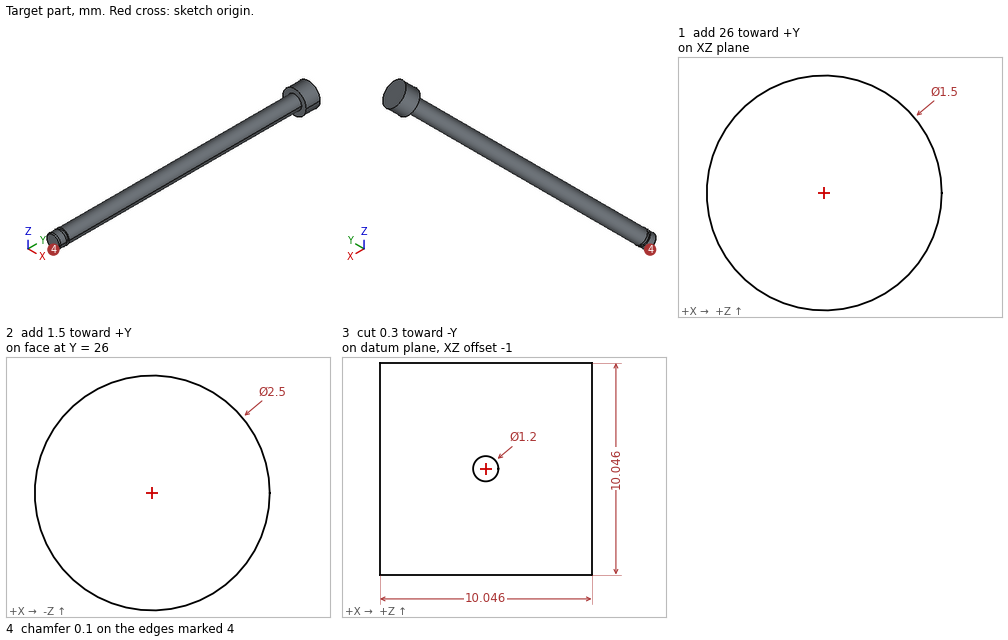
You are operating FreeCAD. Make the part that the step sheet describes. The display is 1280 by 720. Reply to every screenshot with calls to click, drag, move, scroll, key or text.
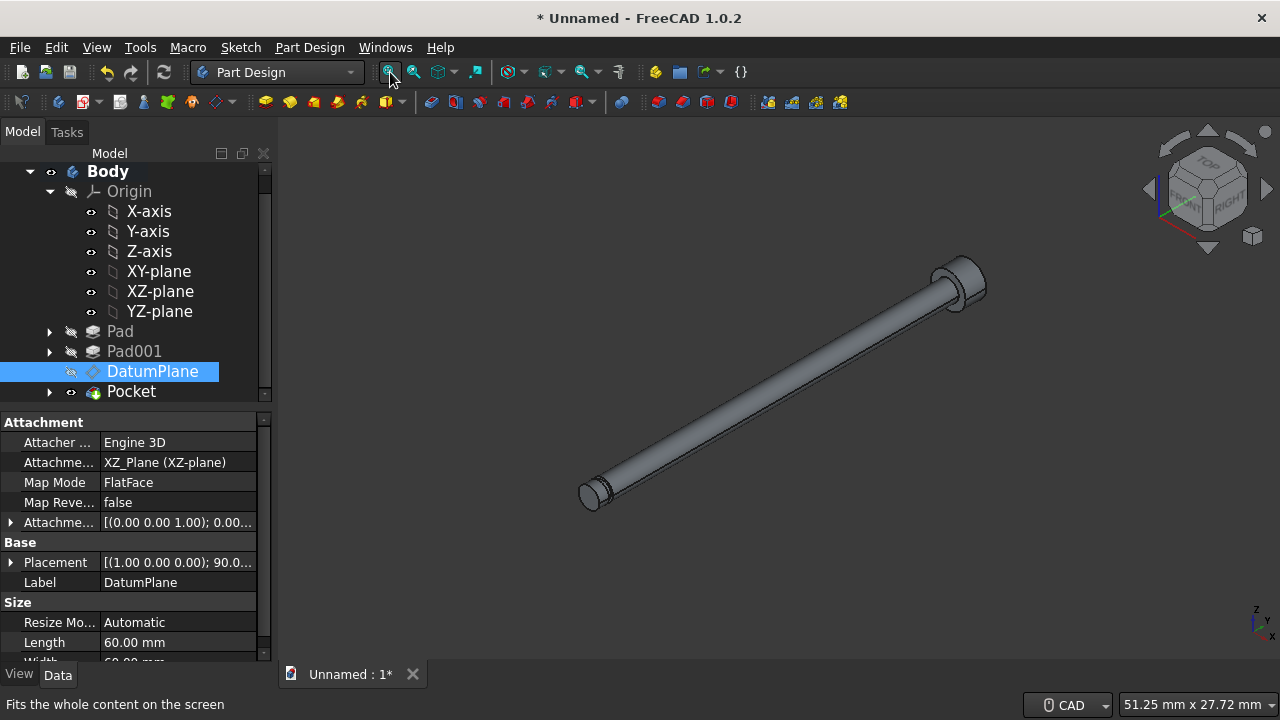
click(581, 485)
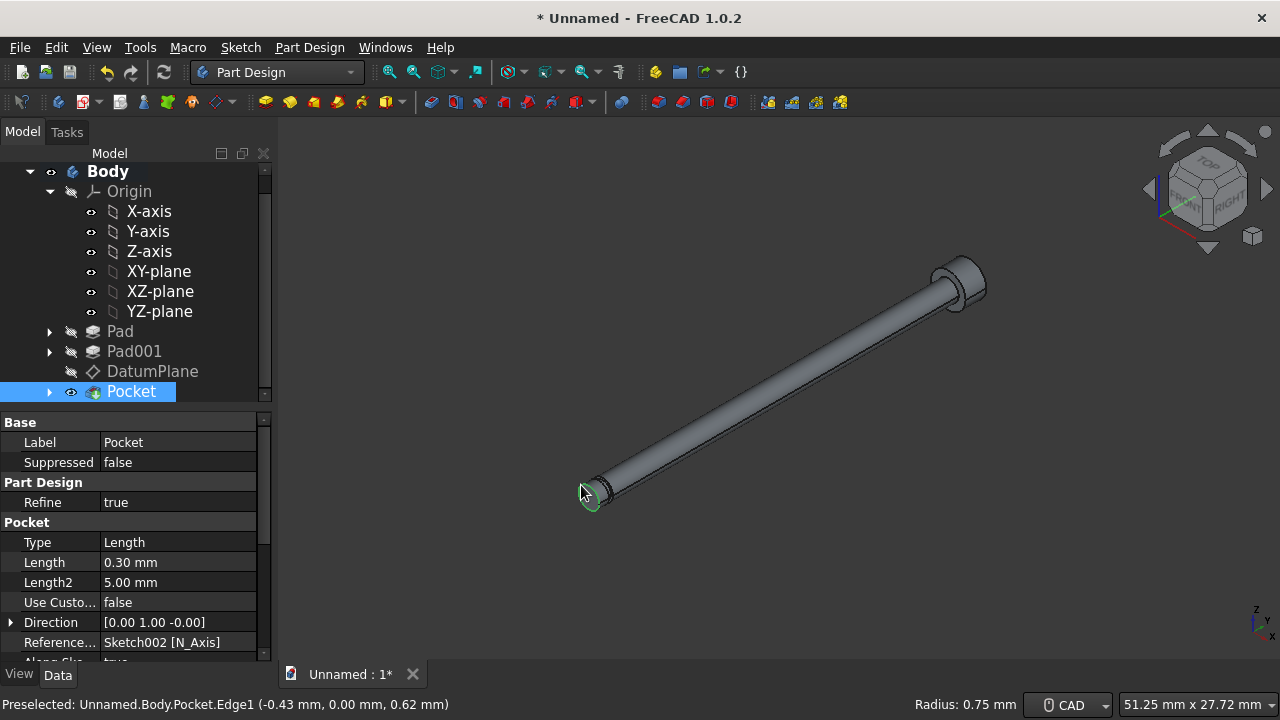
click(684, 102)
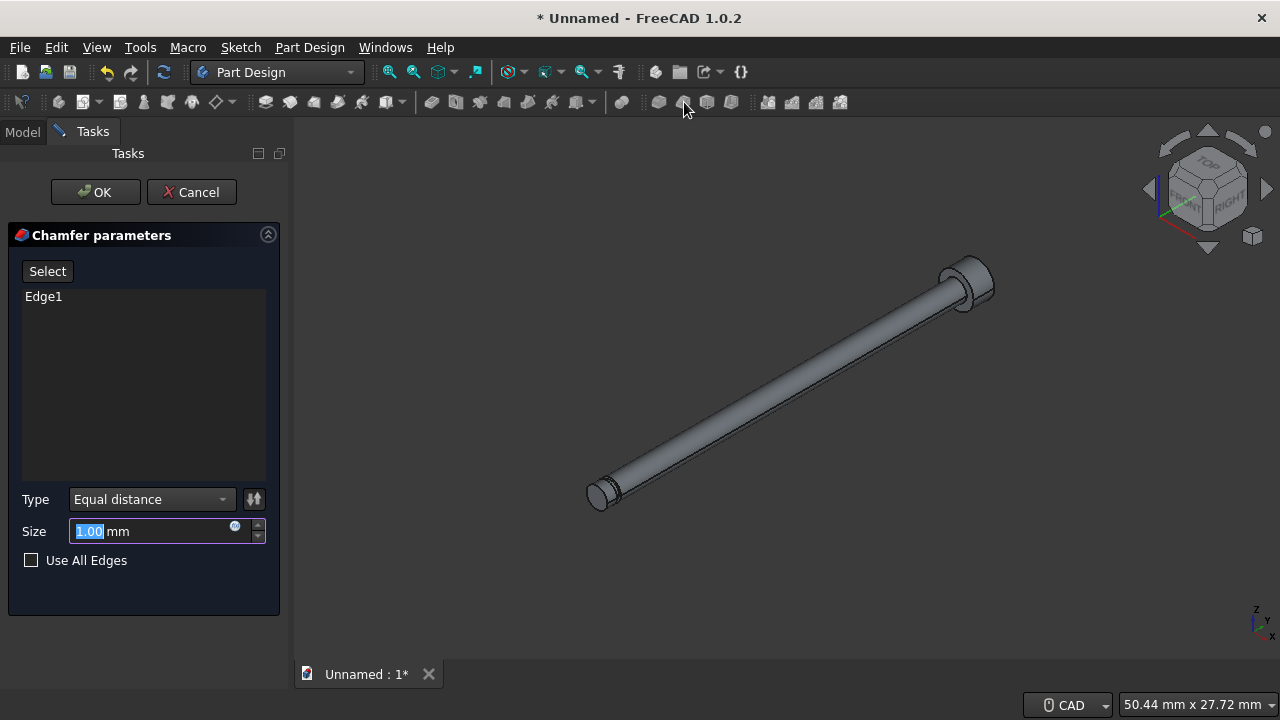
text(0.1)
key(Tab)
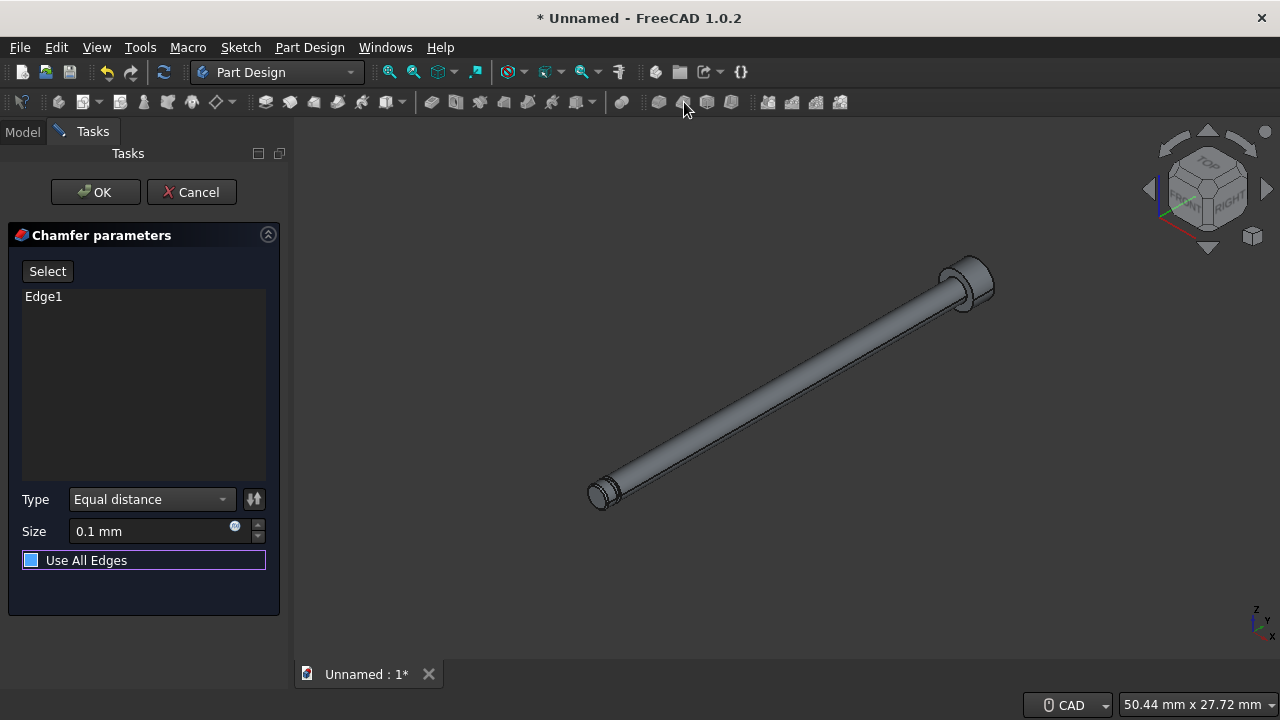
click(96, 192)